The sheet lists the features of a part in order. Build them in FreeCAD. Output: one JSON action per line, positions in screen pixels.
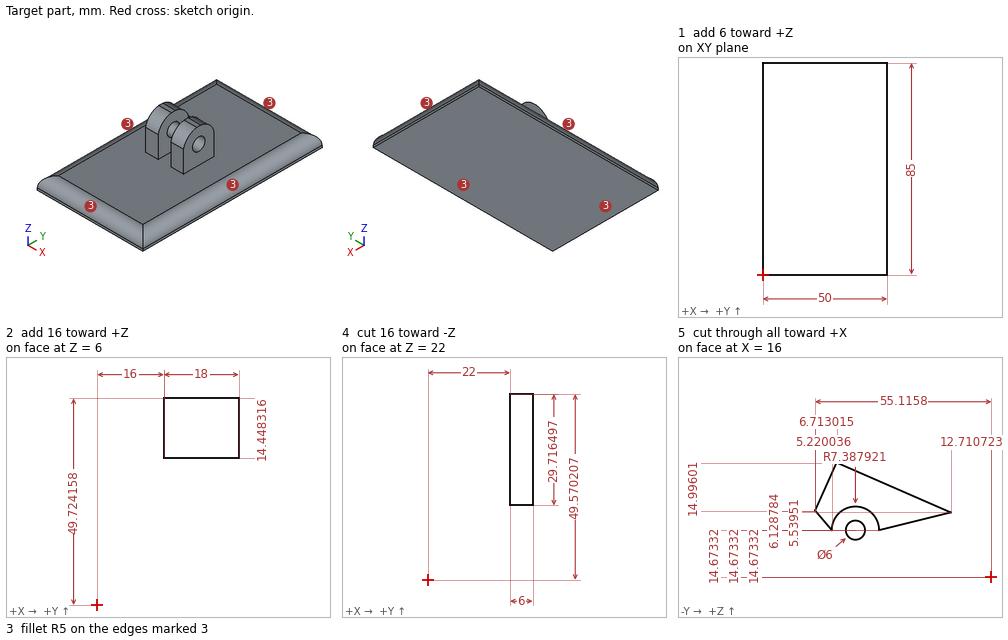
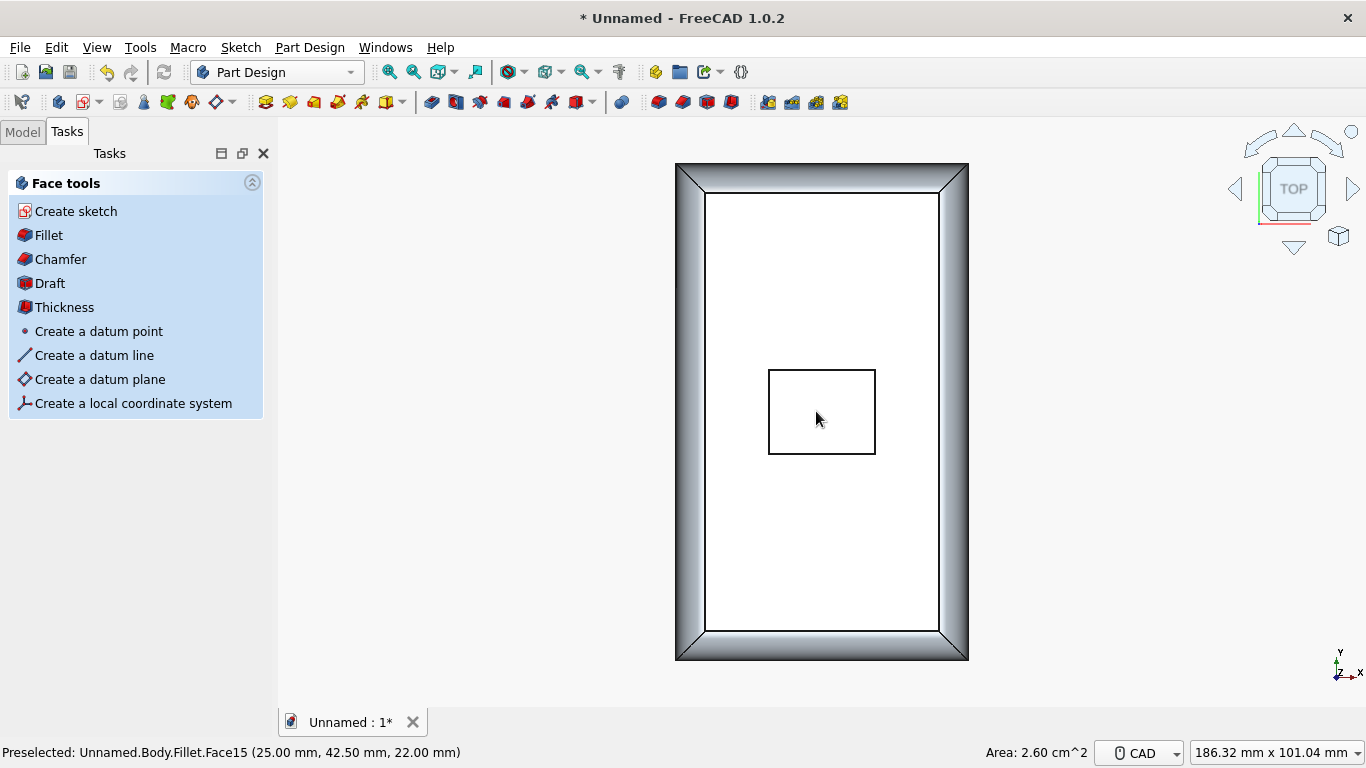
{"action": "left_click", "coordinate": [84, 102]}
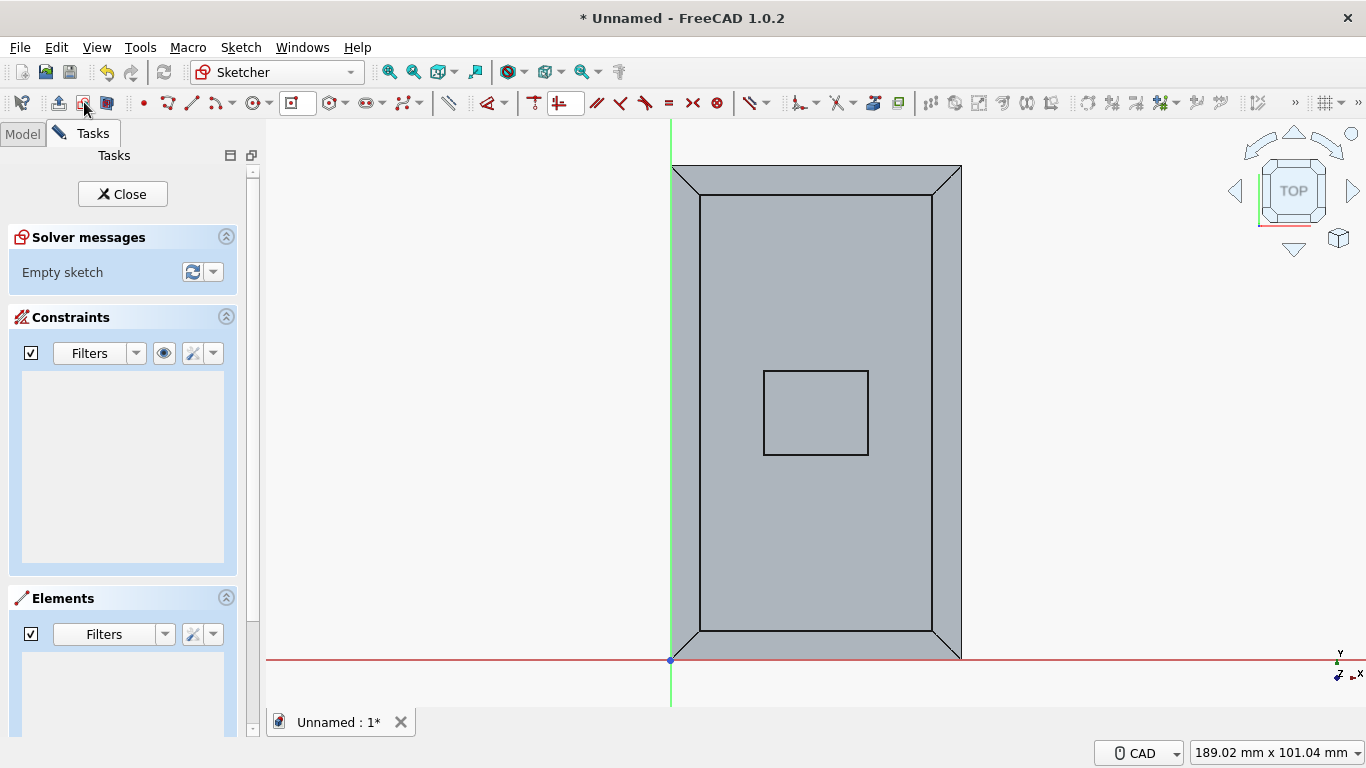
{"action": "scroll", "coordinate": [727, 147], "scroll_direction": "down", "scroll_amount": 1}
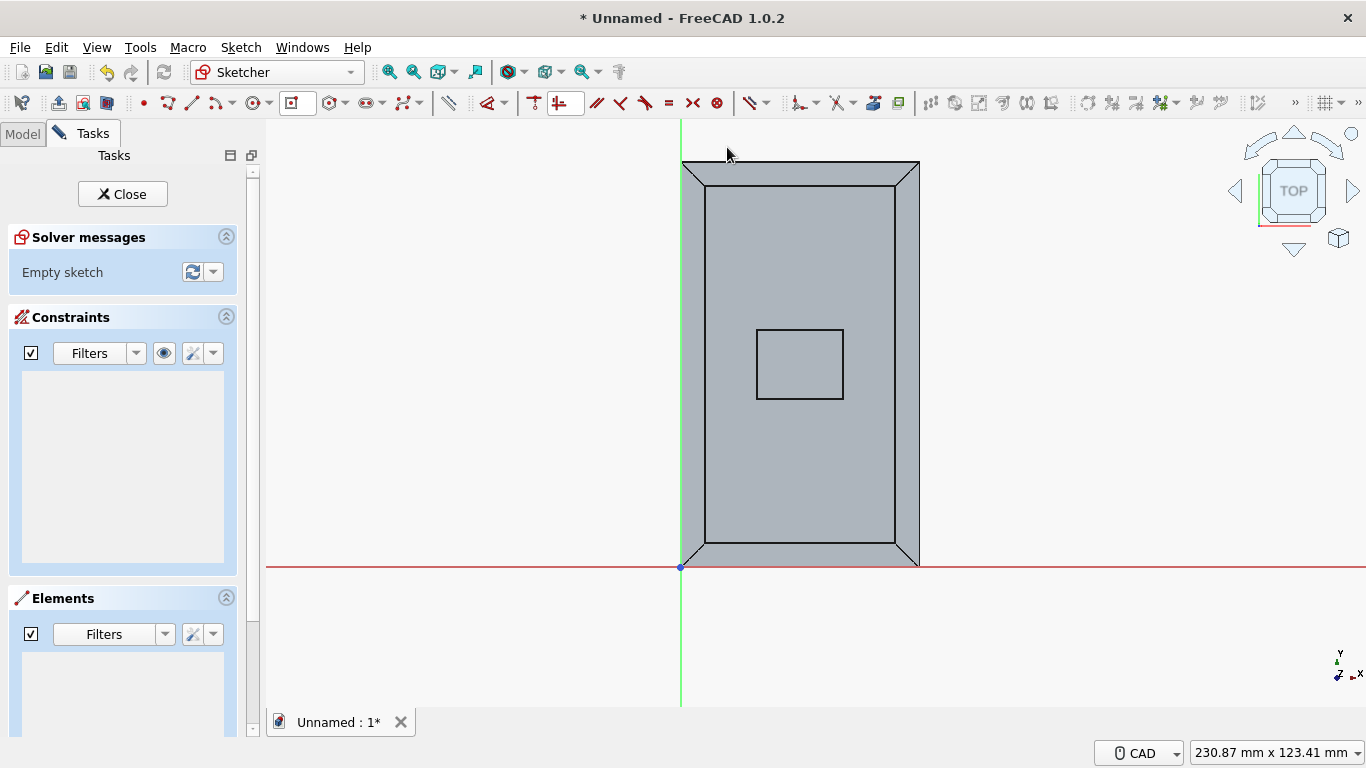
{"action": "scroll", "coordinate": [748, 523], "scroll_direction": "up", "scroll_amount": 2}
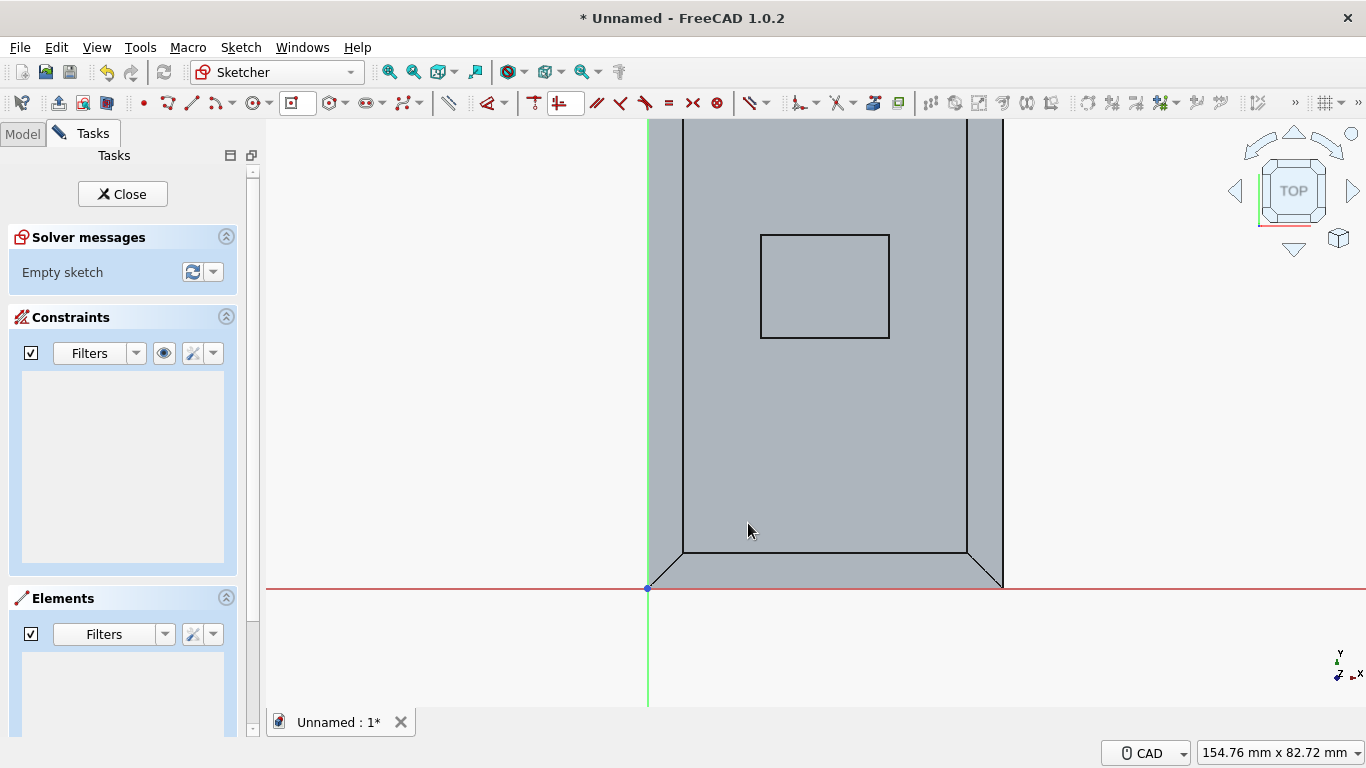
{"action": "left_click", "coordinate": [310, 104]}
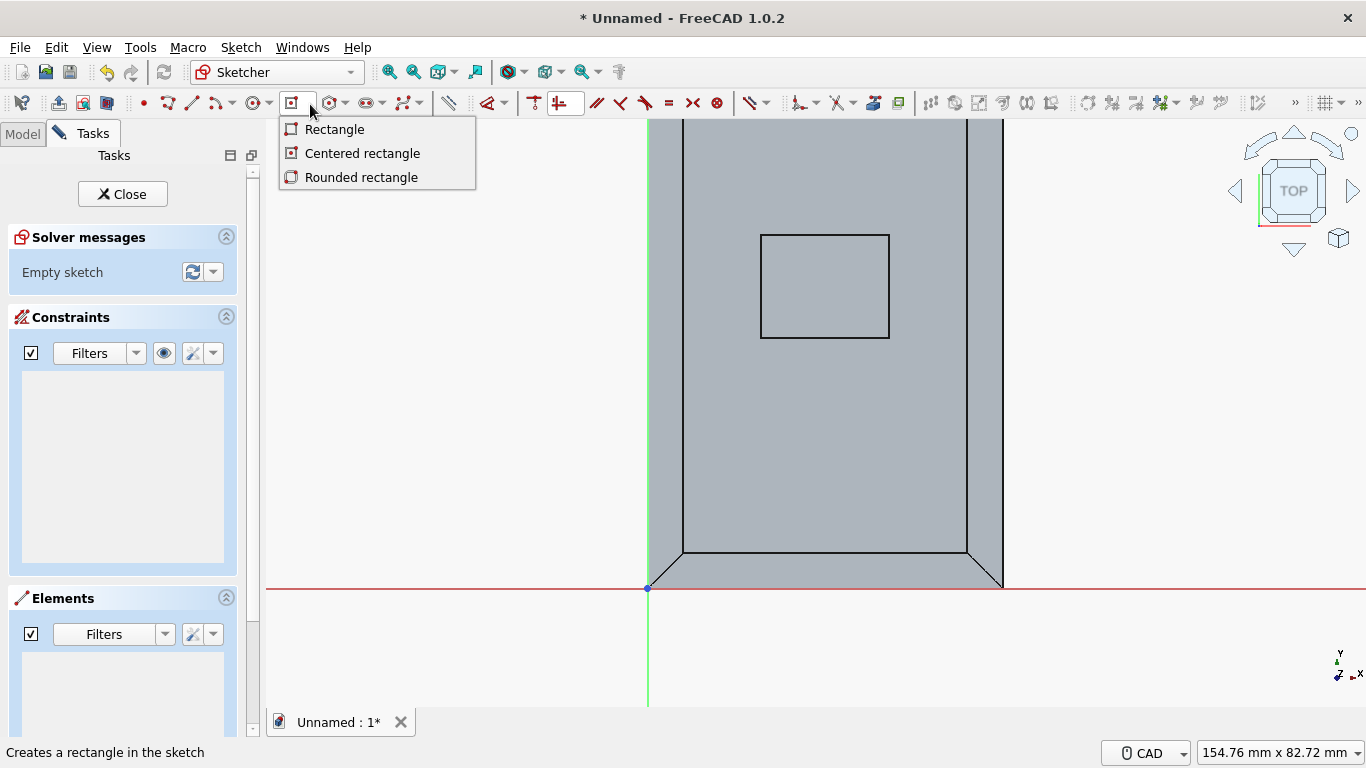
{"action": "left_click", "coordinate": [378, 129]}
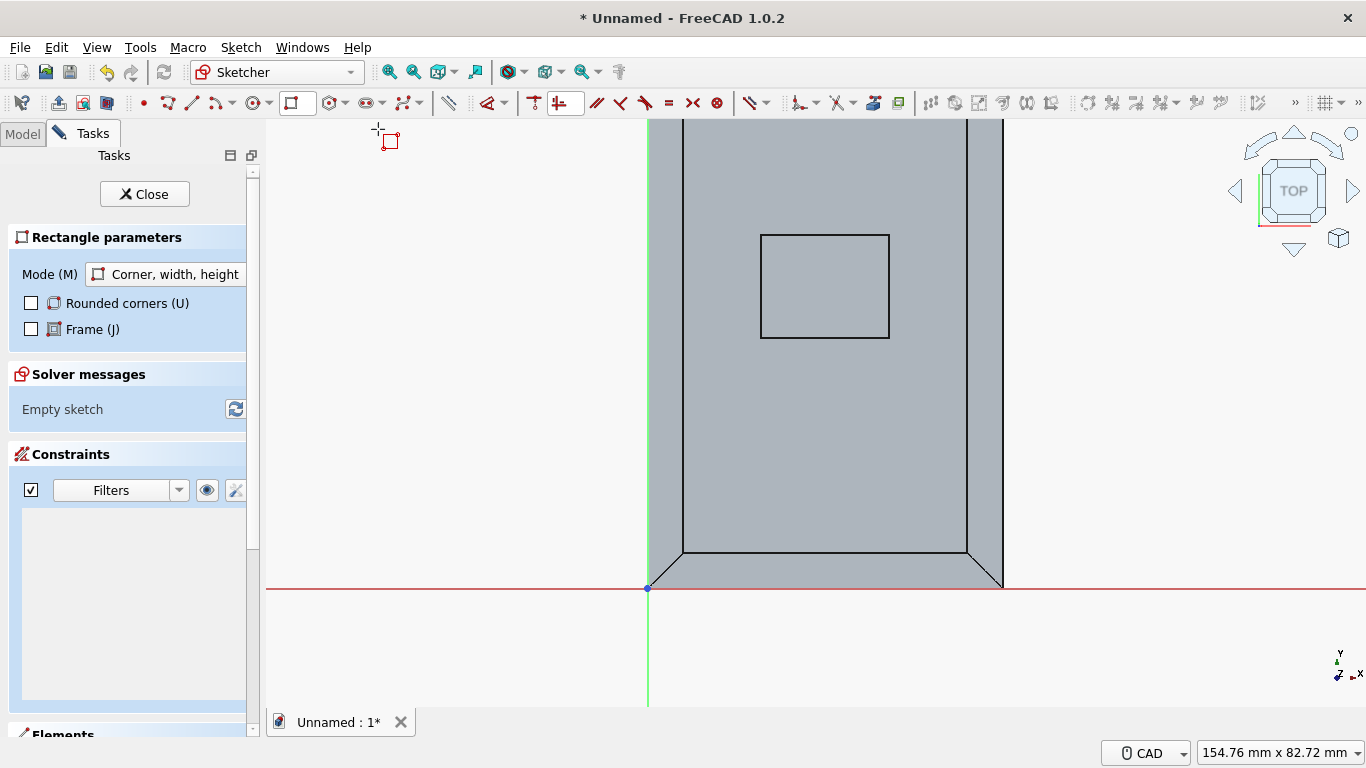
{"action": "left_click", "coordinate": [804, 236]}
{"action": "mouse_move", "coordinate": [847, 448]}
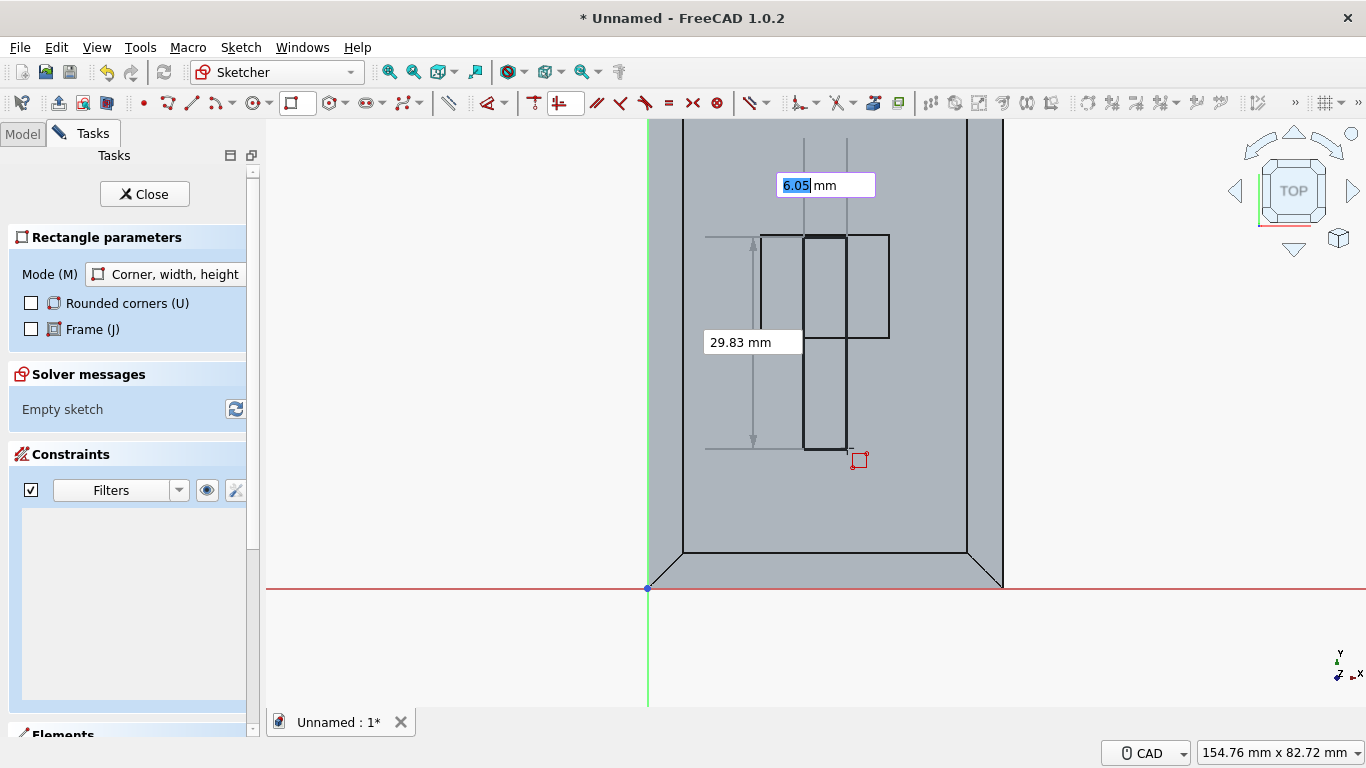
{"action": "type", "text": "6"}
{"action": "key", "text": "Tab"}
{"action": "type", "text": "29.716497"}
{"action": "key", "text": "Return"}
{"action": "key", "text": "Escape"}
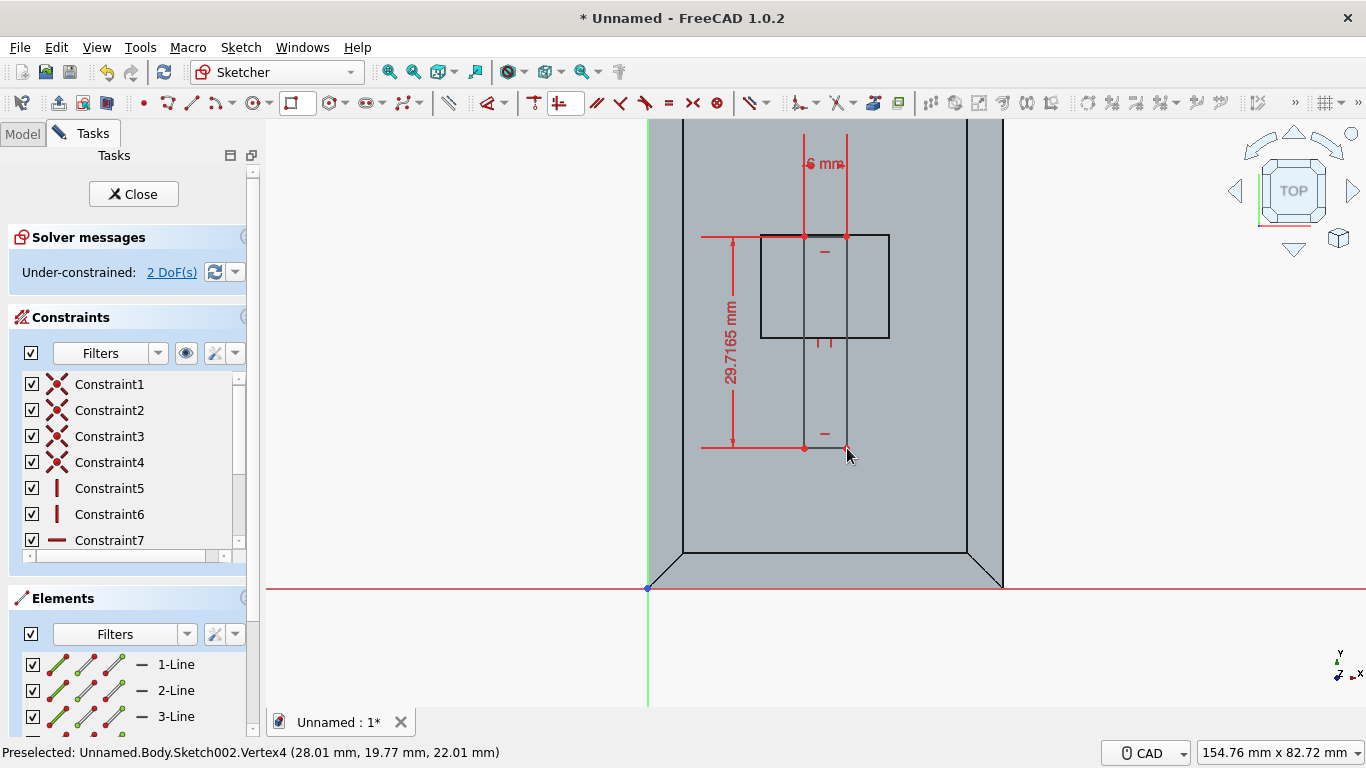
{"action": "key", "text": "d"}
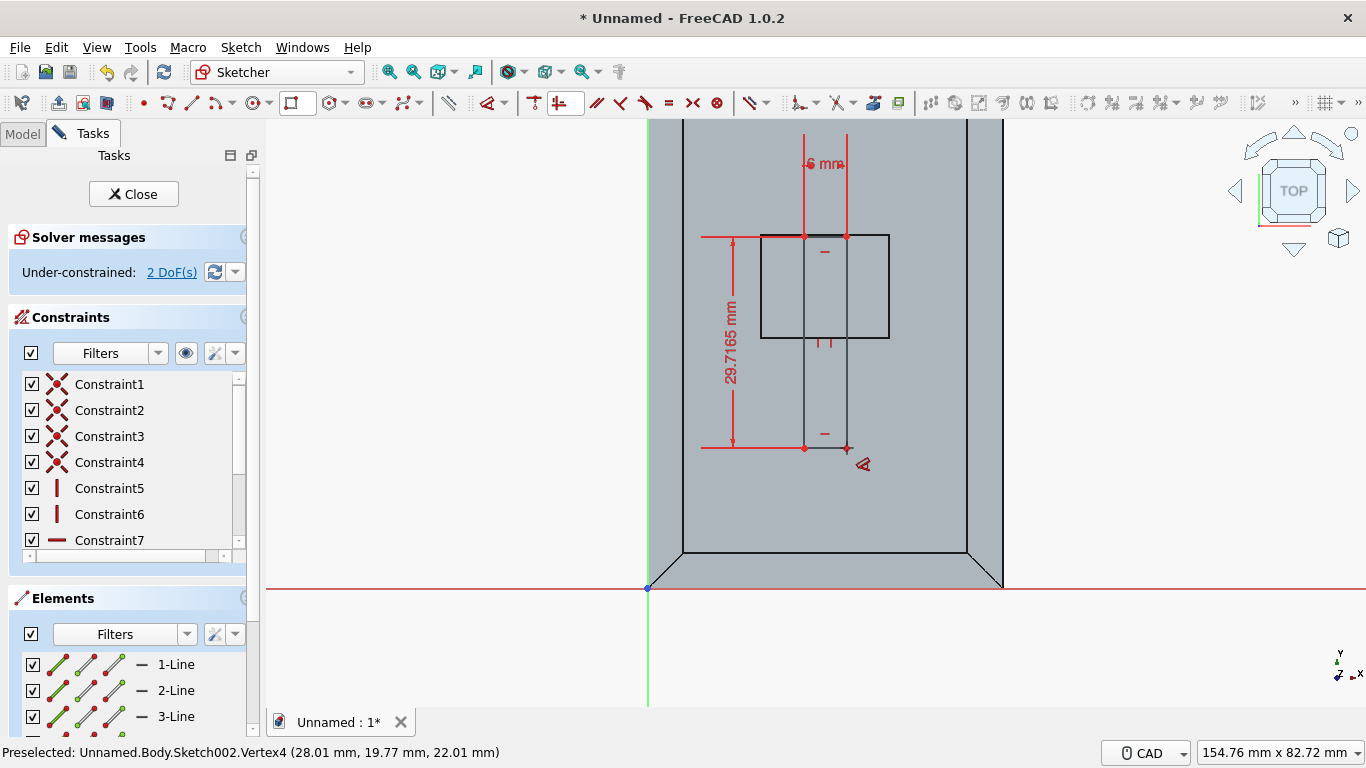
{"action": "left_click", "coordinate": [804, 237]}
{"action": "left_click", "coordinate": [726, 623]}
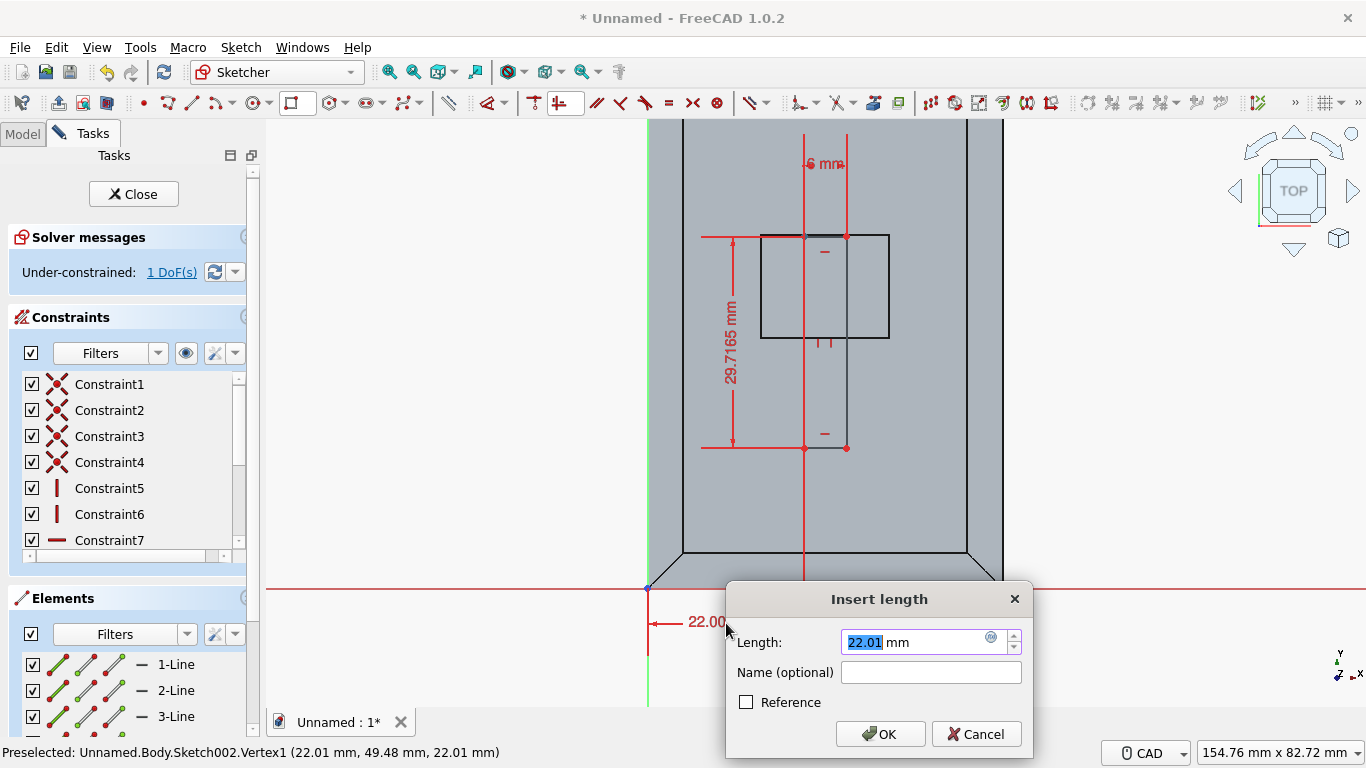
{"action": "type", "text": "22"}
{"action": "key", "text": "Return"}